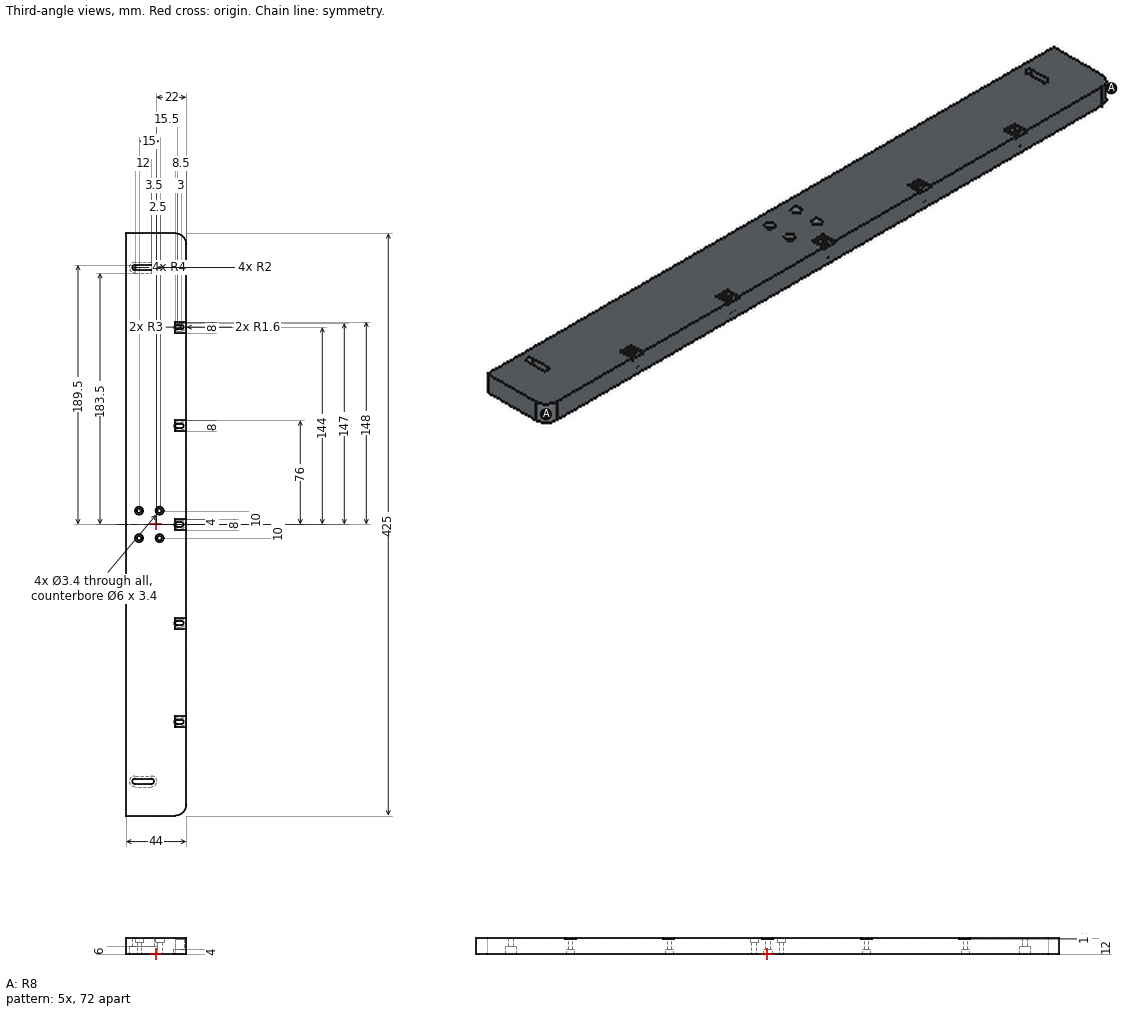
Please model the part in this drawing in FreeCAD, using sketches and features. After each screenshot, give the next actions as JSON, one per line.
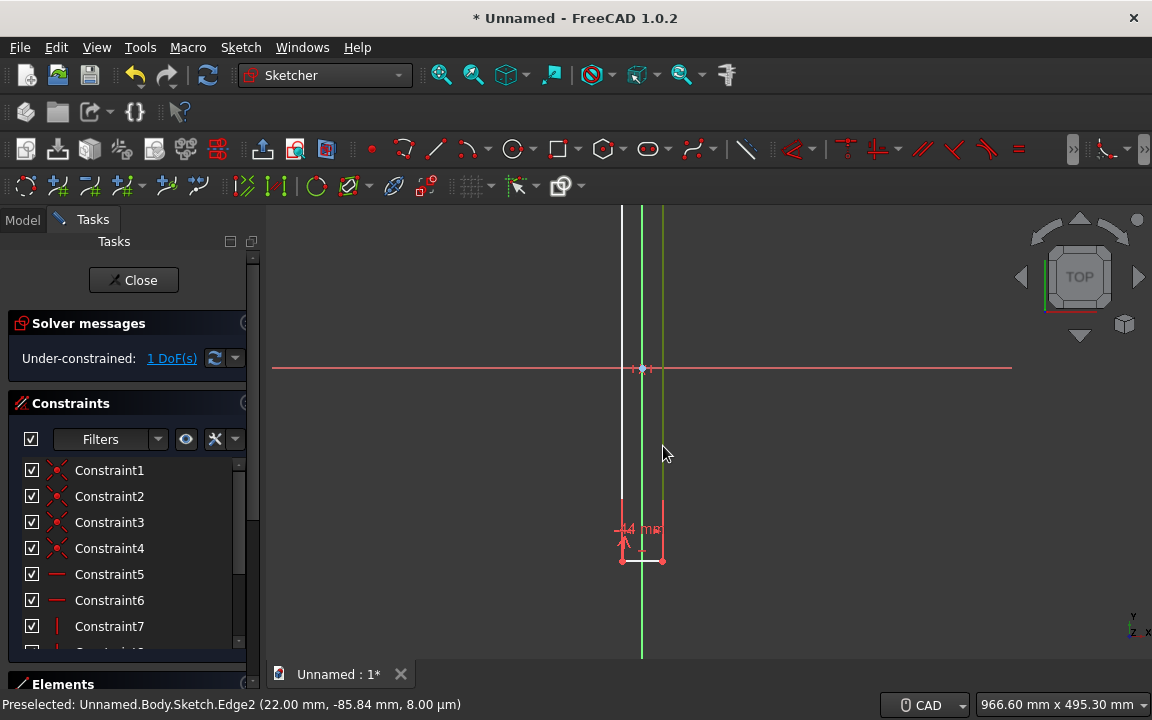
{"action": "key", "text": "i"}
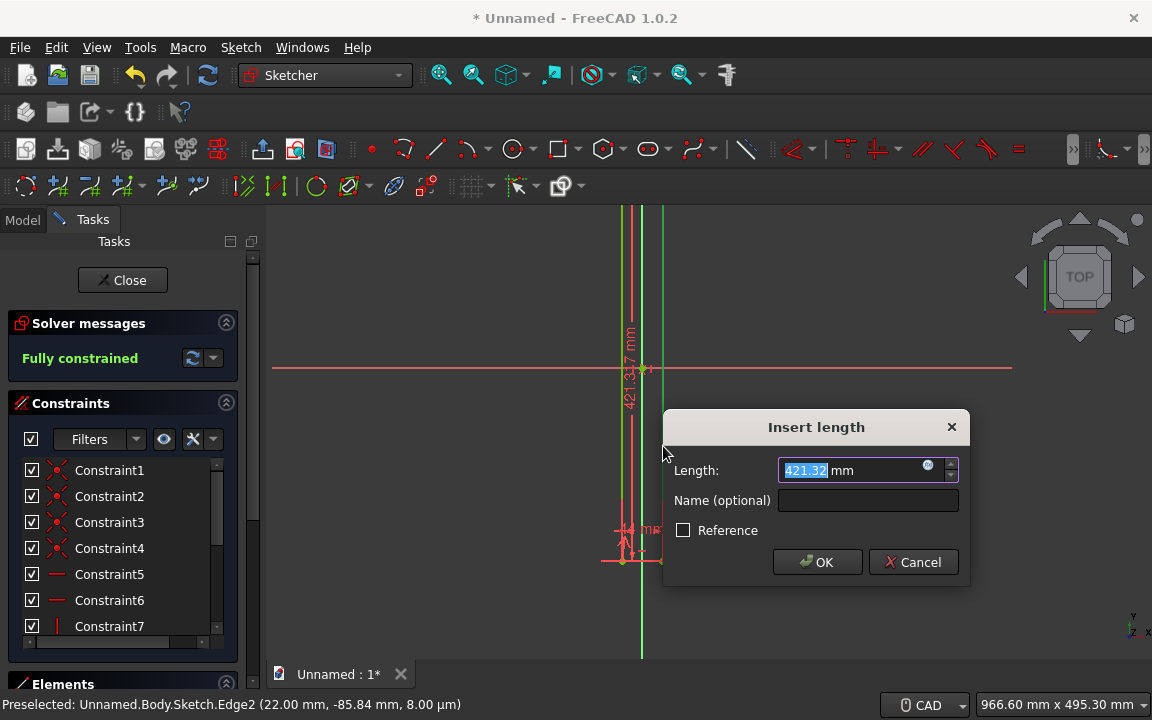
{"action": "type", "text": "425"}
{"action": "key", "text": "Return"}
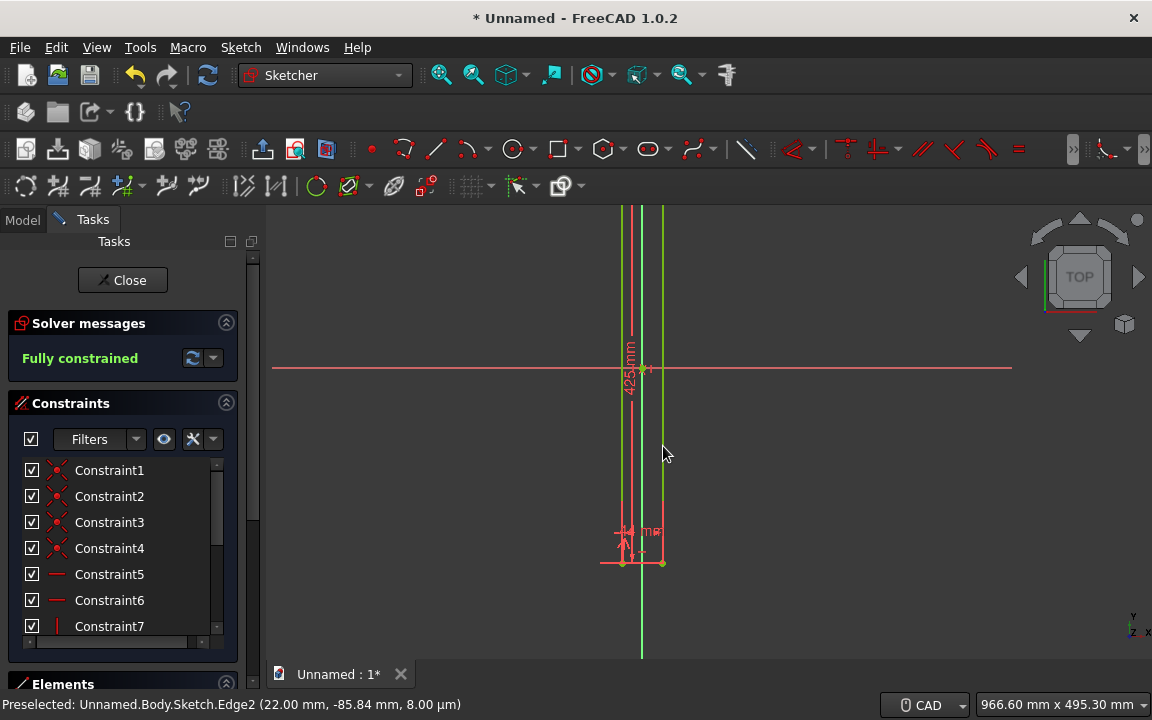
{"action": "left_click", "coordinate": [123, 280]}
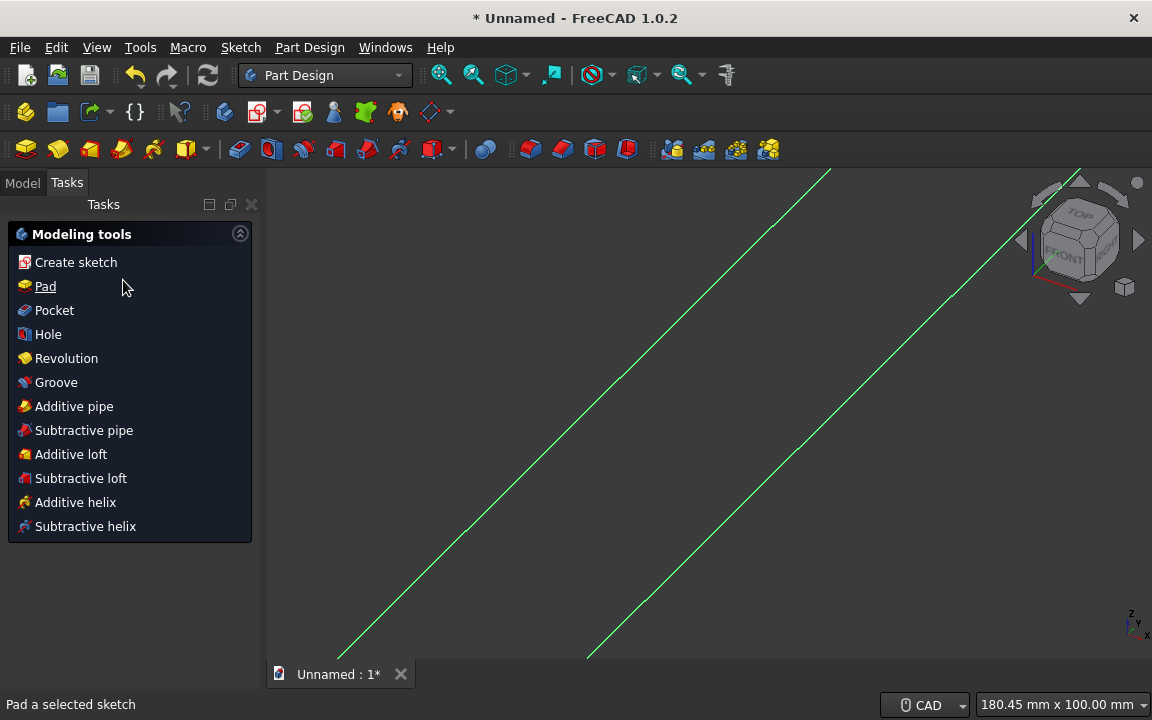
{"action": "left_click", "coordinate": [26, 150]}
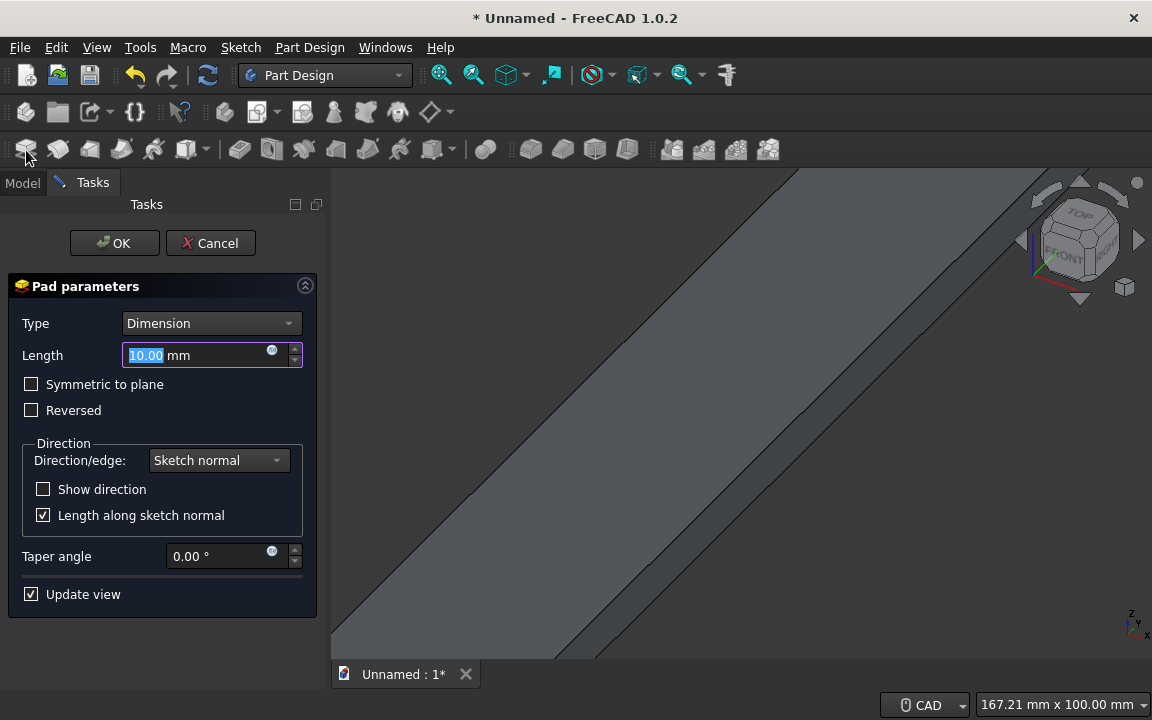
{"action": "type", "text": "12"}
{"action": "key", "text": "Tab"}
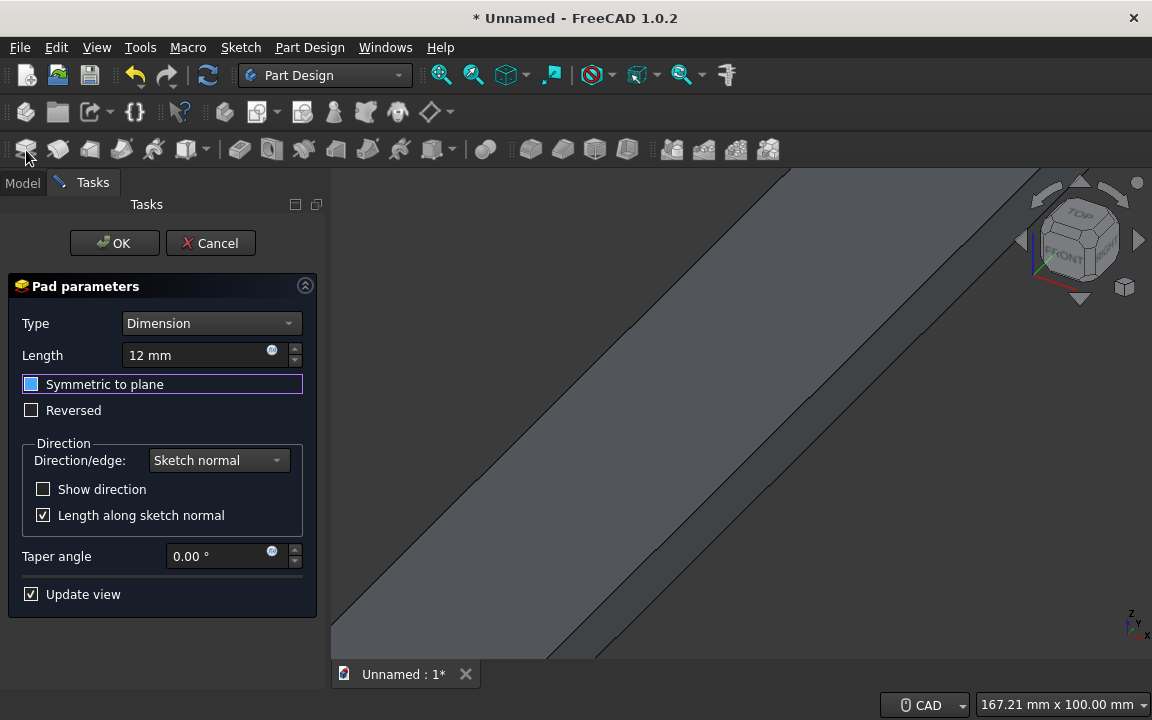
{"action": "left_click", "coordinate": [115, 243]}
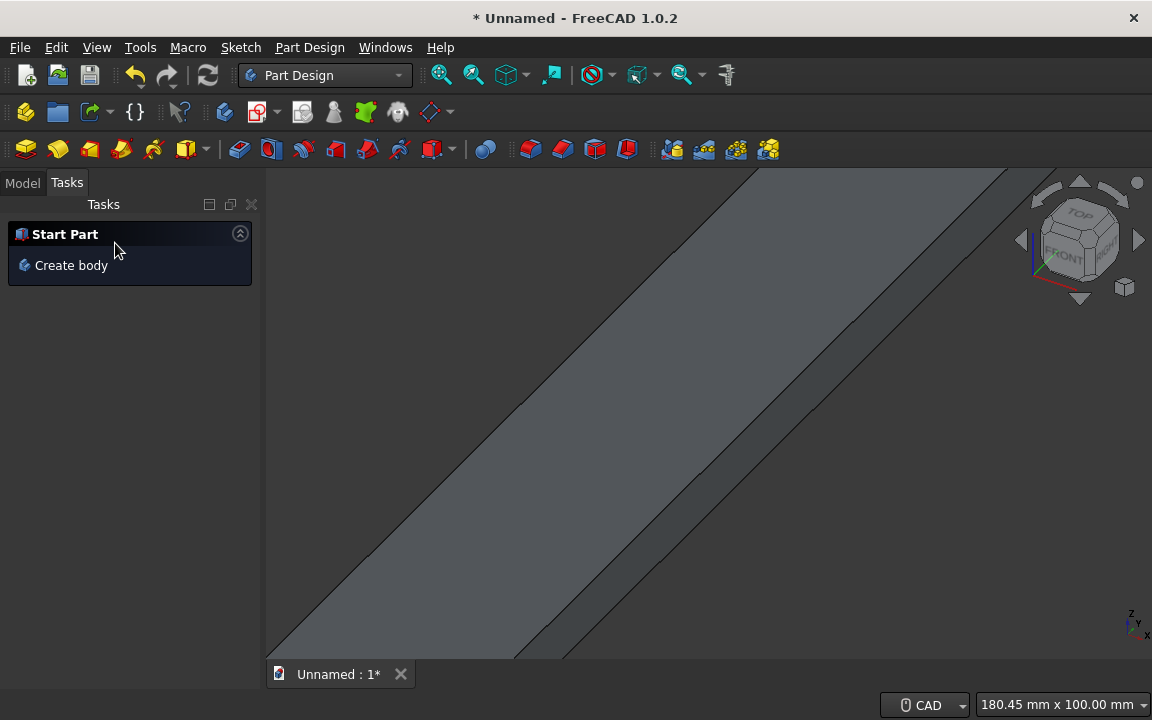
{"action": "key", "text": "v f"}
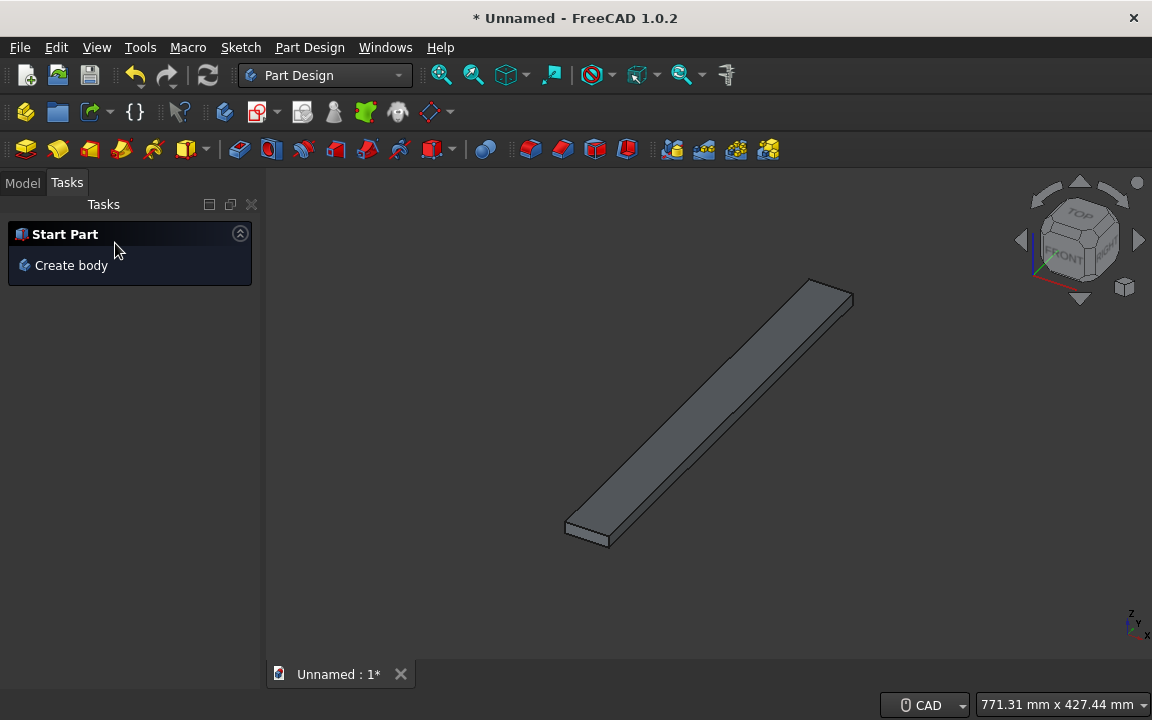
{"action": "left_click", "coordinate": [609, 542]}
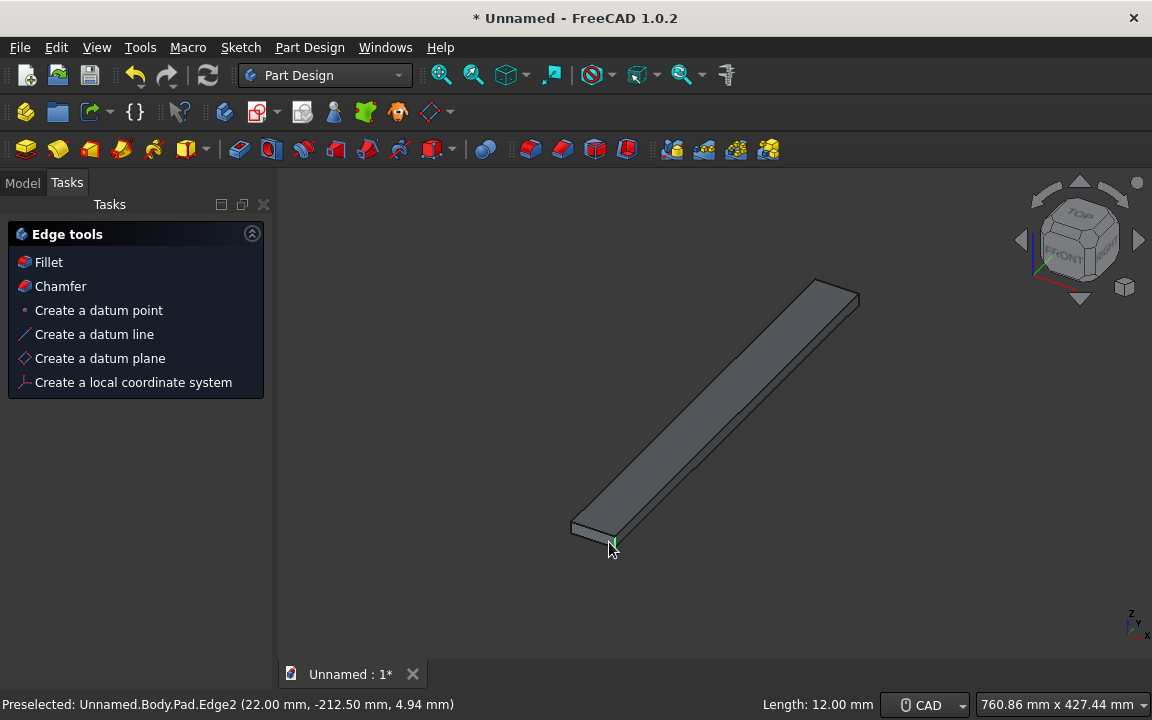
{"action": "scroll", "coordinate": [859, 298], "scroll_direction": "up", "scroll_amount": 6}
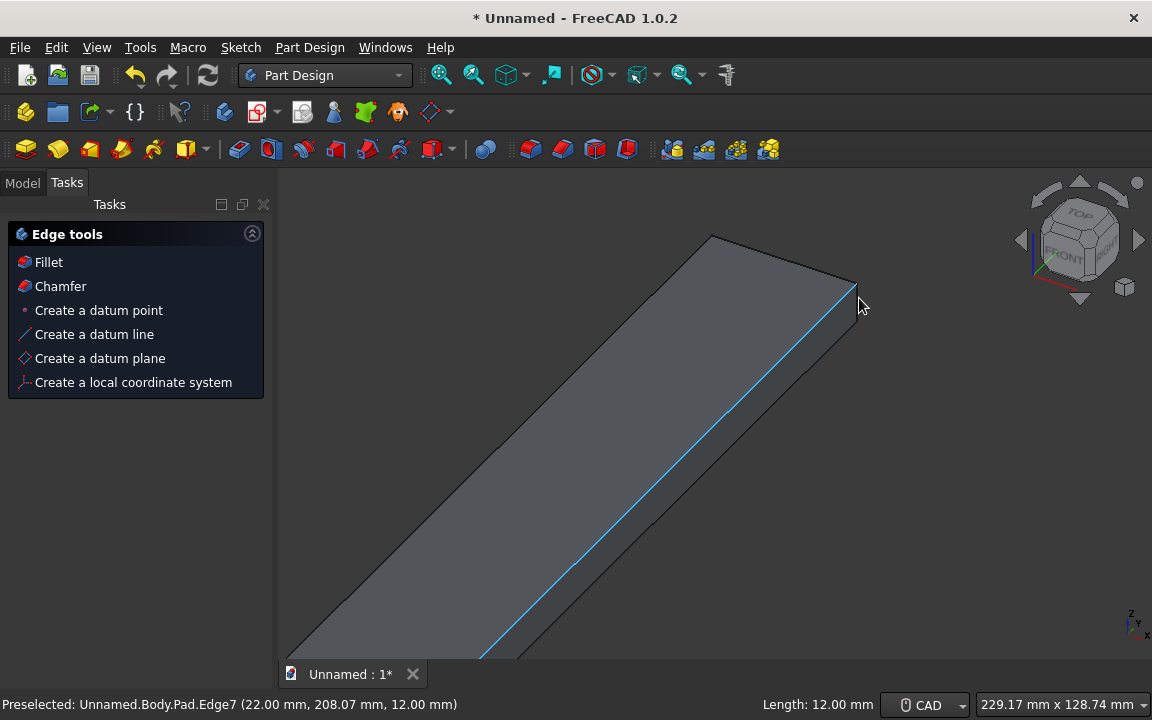
{"action": "left_click", "coordinate": [442, 76]}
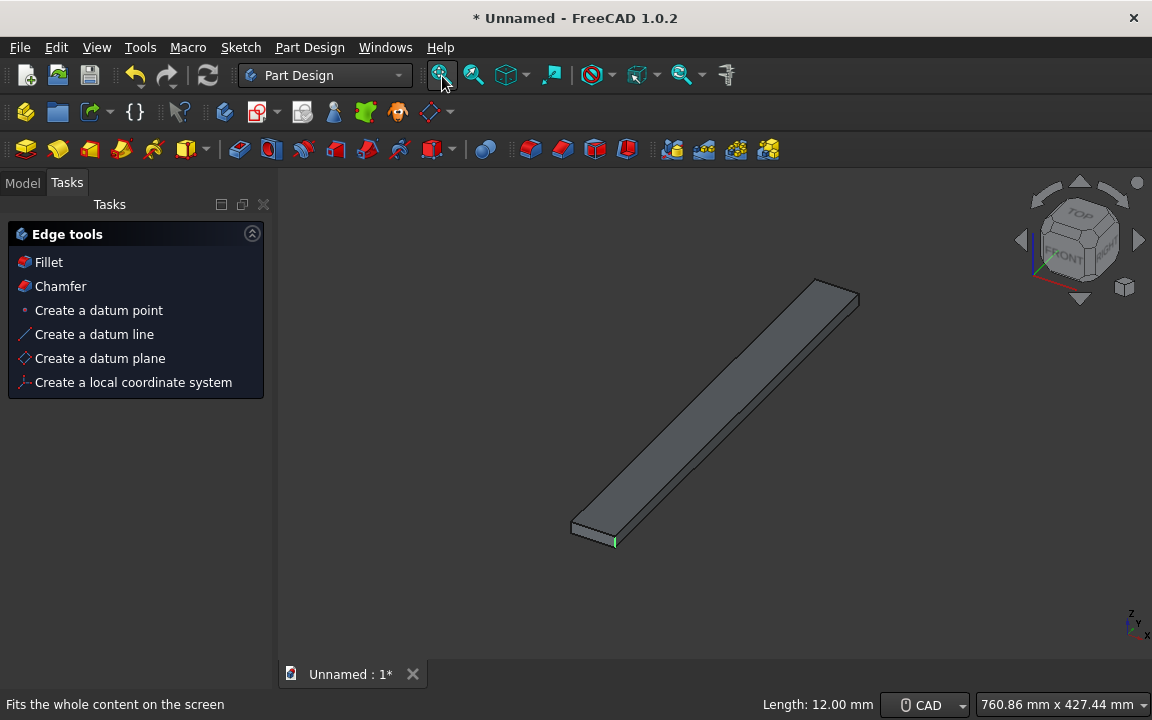
{"action": "key", "text": "0"}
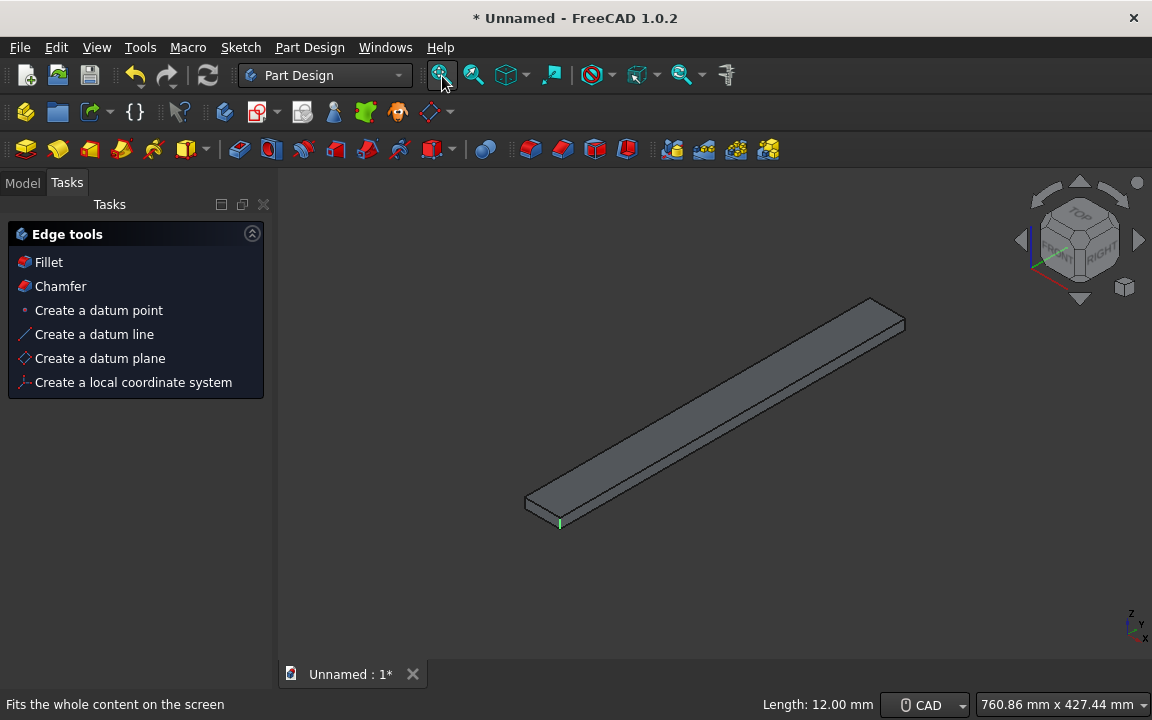
{"action": "scroll", "coordinate": [905, 323], "scroll_direction": "up", "scroll_amount": 6}